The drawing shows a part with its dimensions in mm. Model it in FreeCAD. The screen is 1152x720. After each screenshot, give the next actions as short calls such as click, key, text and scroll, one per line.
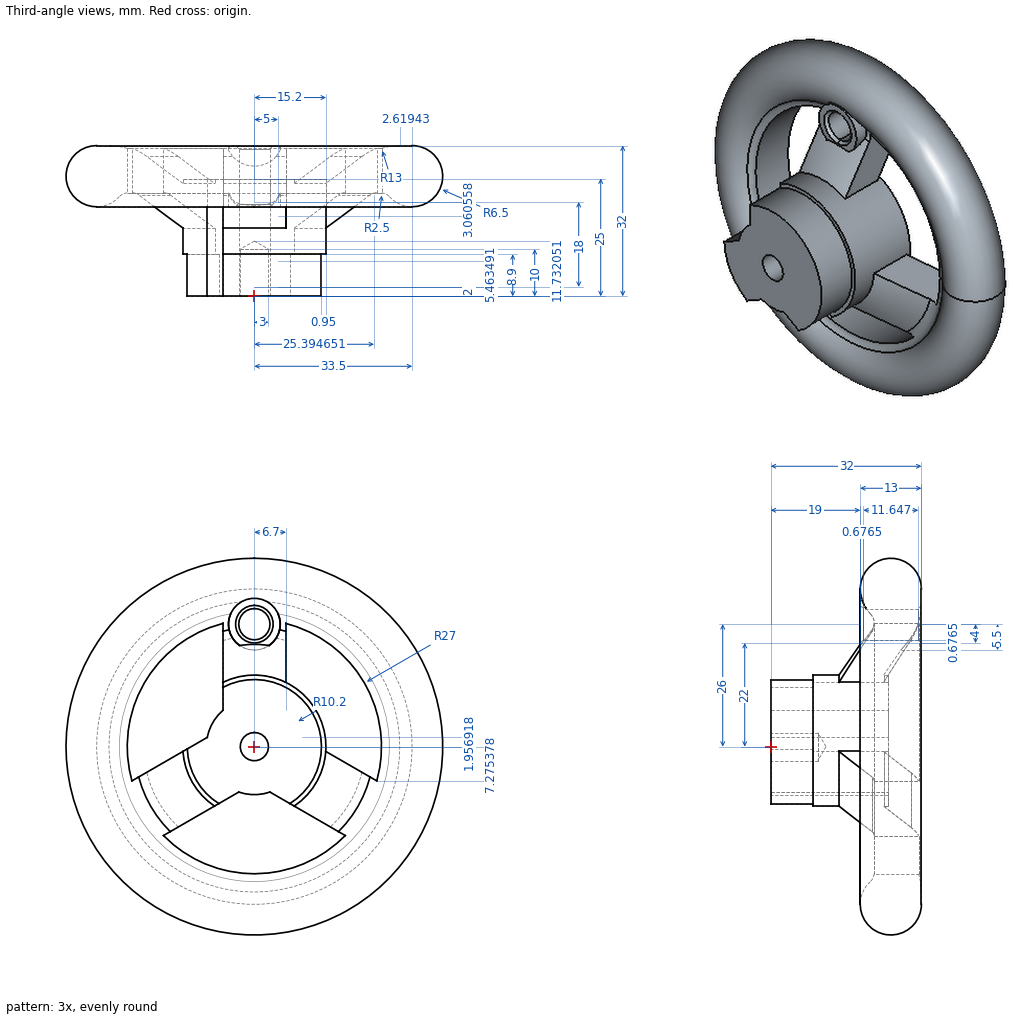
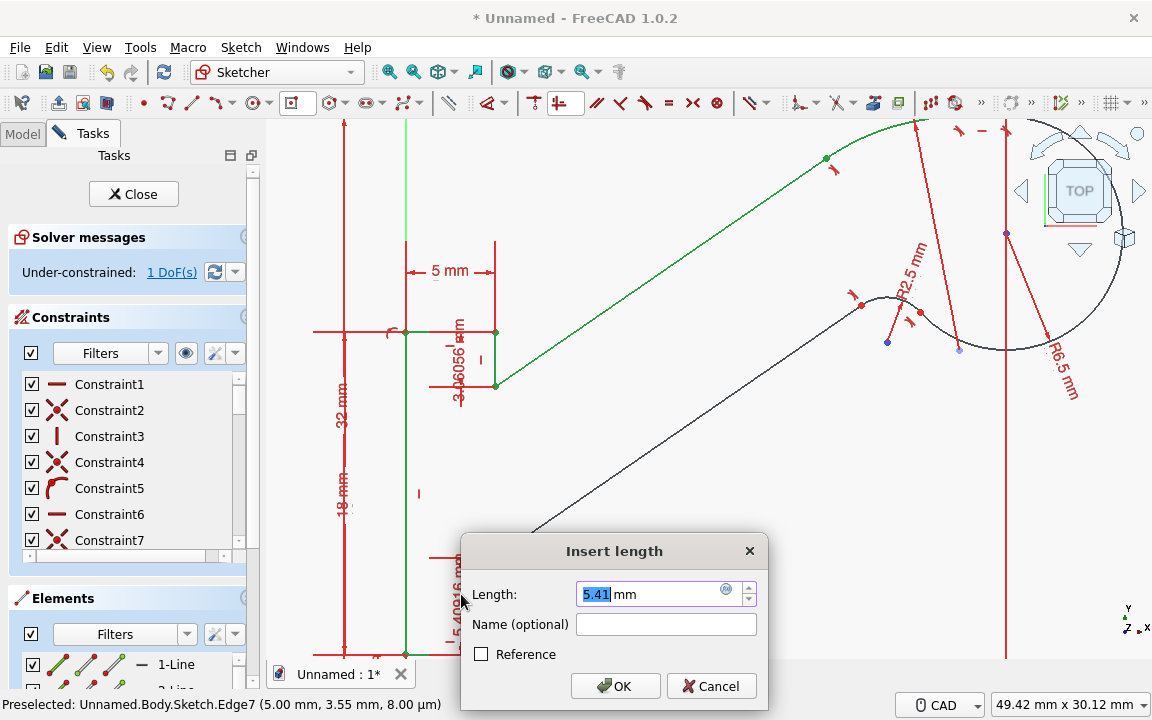
text(5.463491)
key(Return)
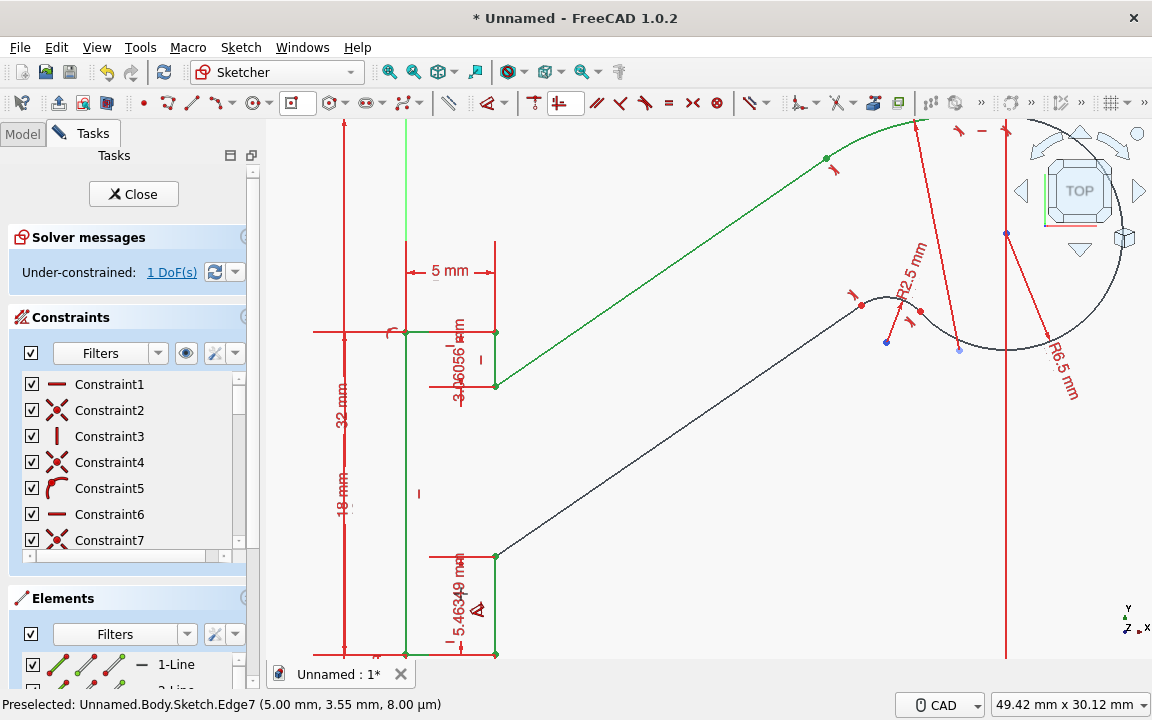
click(862, 305)
click(634, 271)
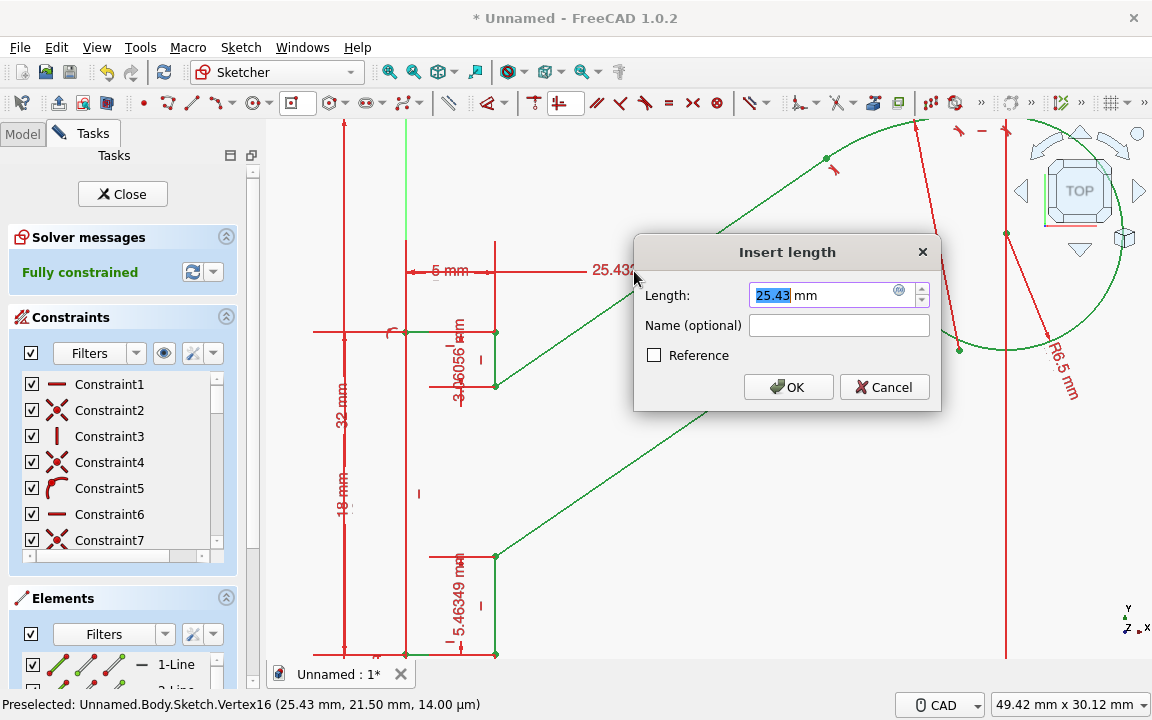
text(25.394651)
key(Return)
key(Escape)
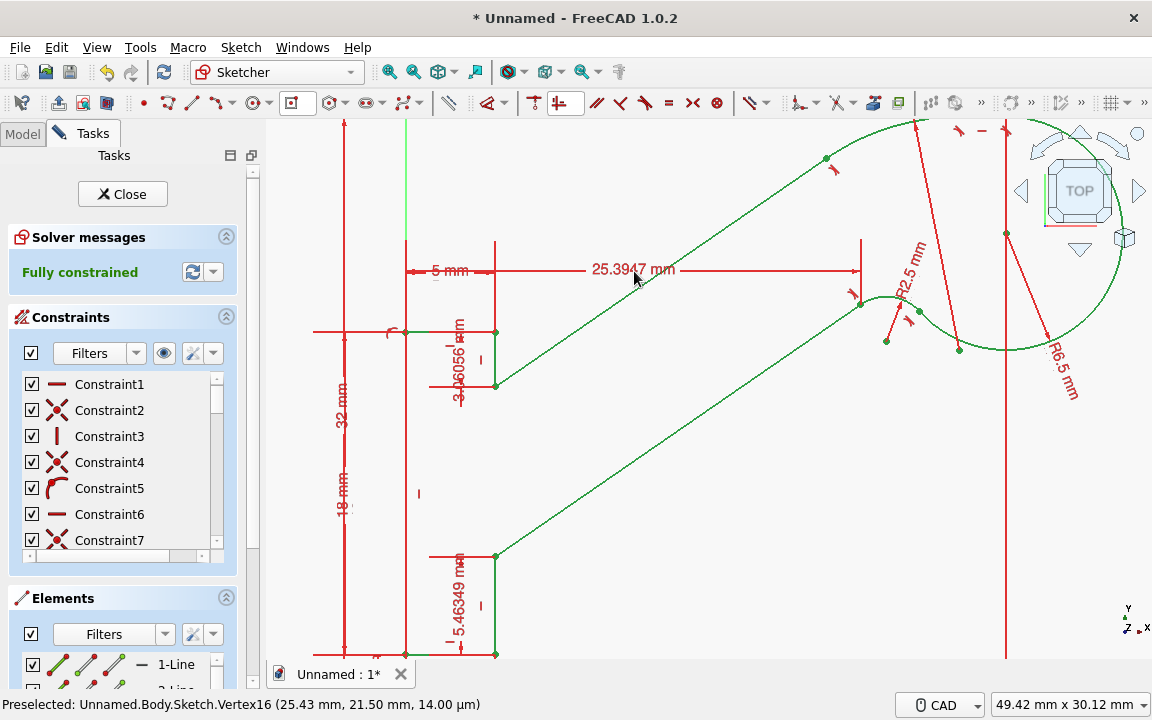
click(123, 194)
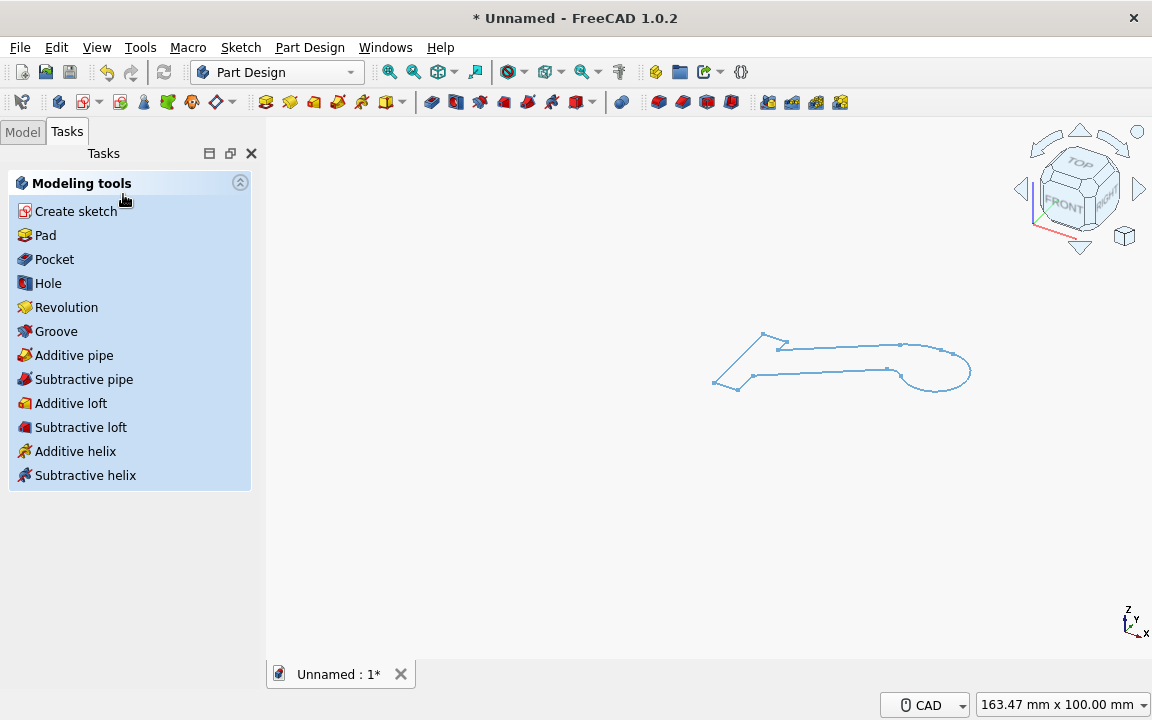
click(290, 102)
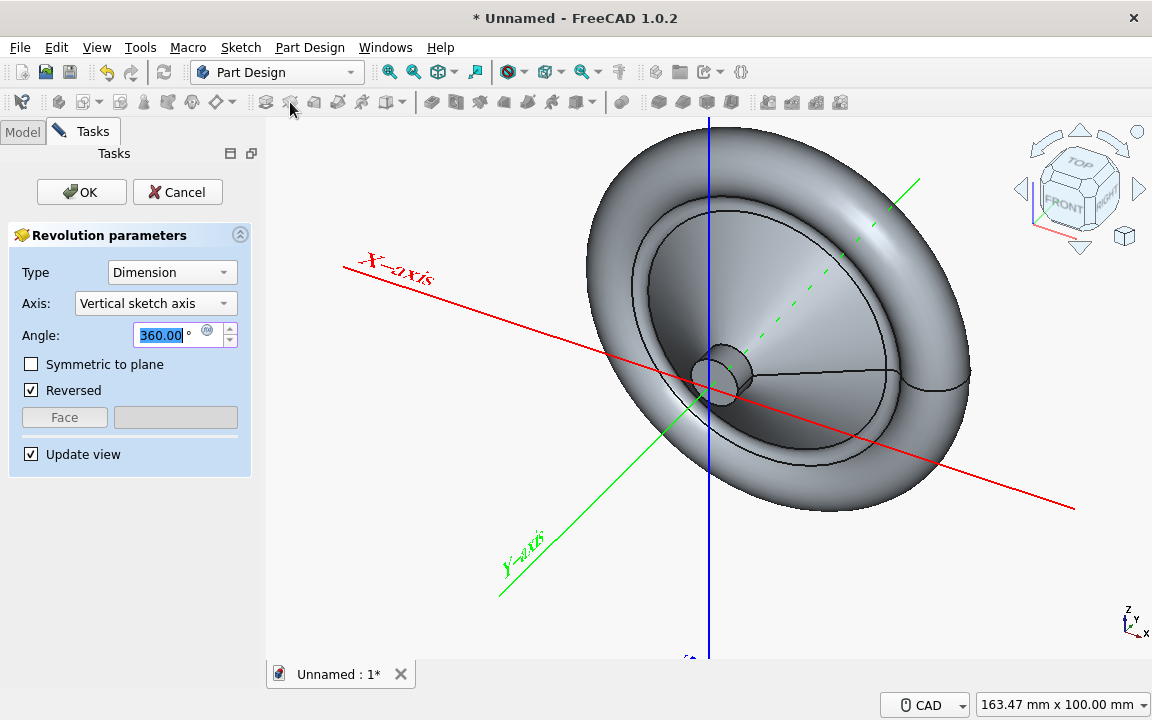
click(82, 192)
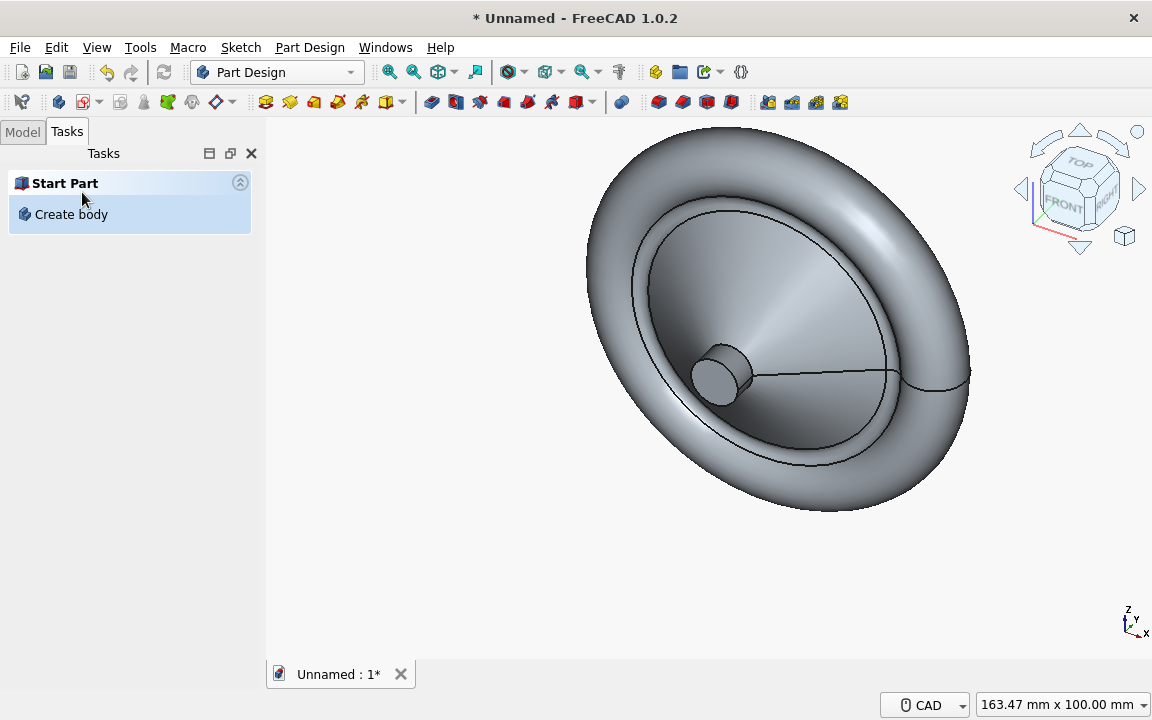
click(390, 72)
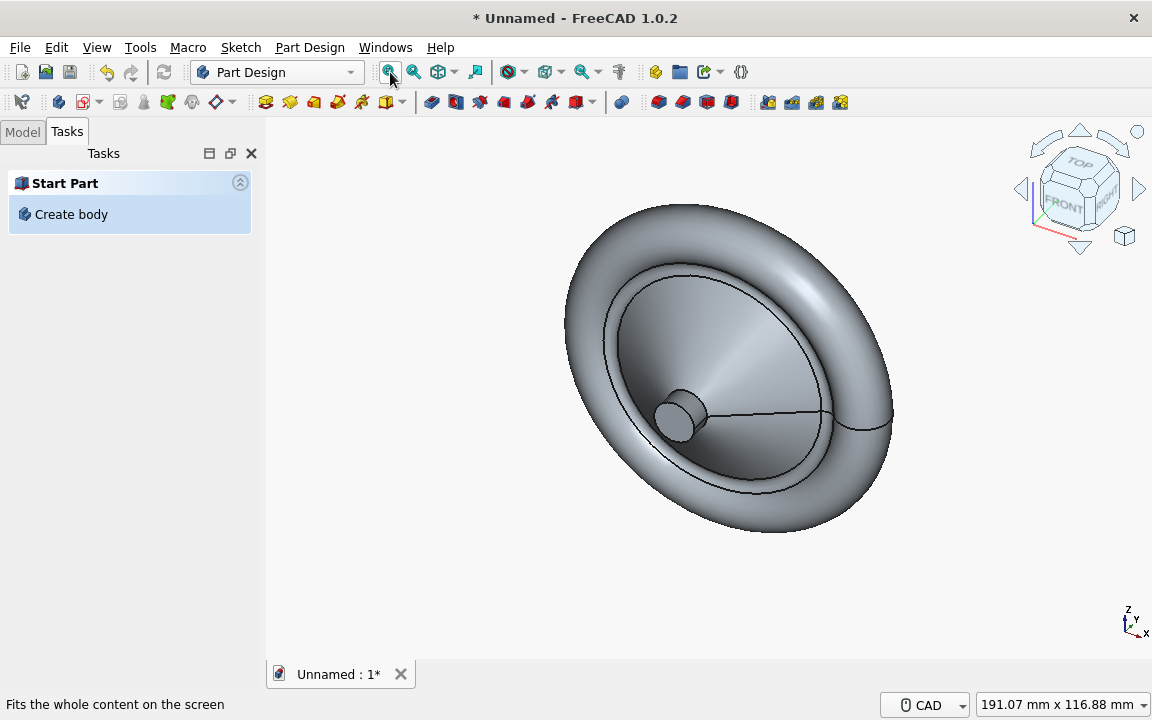
click(84, 102)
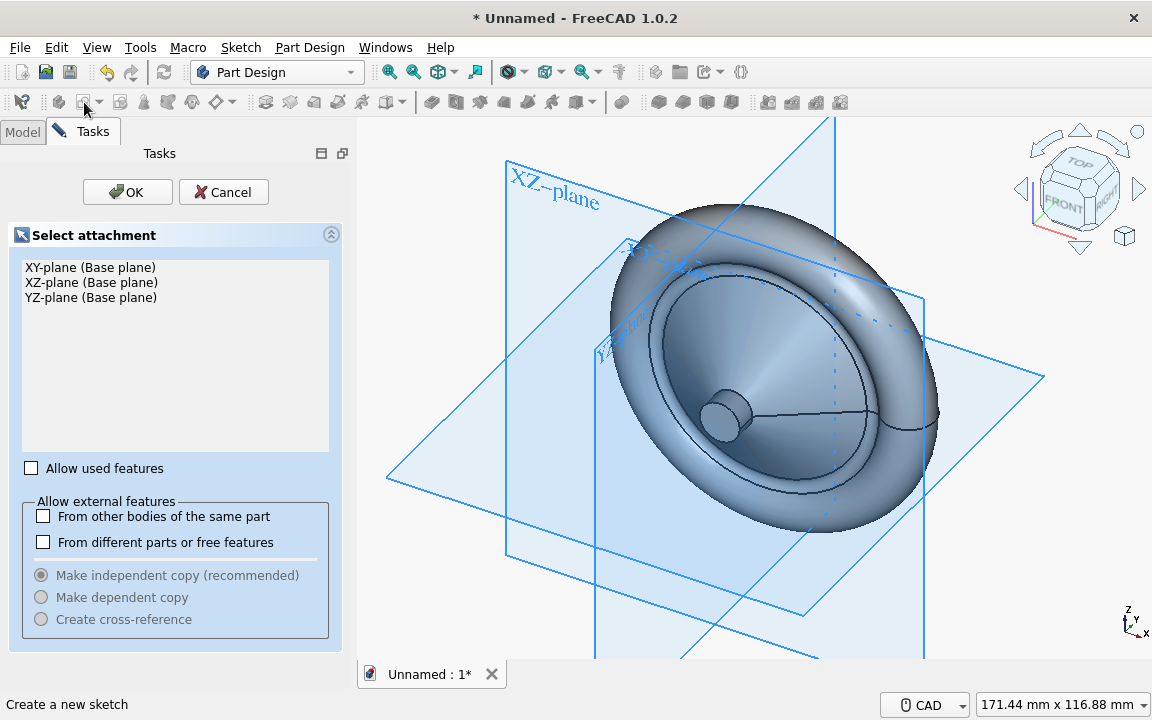
click(82, 282)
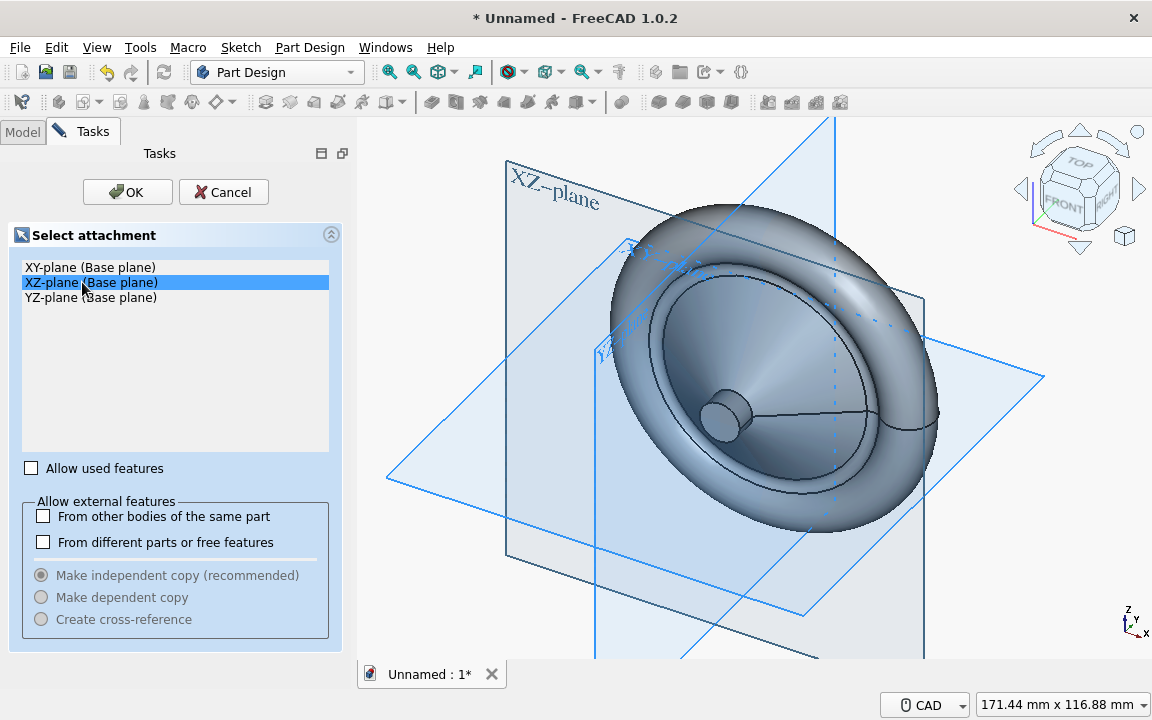
click(128, 192)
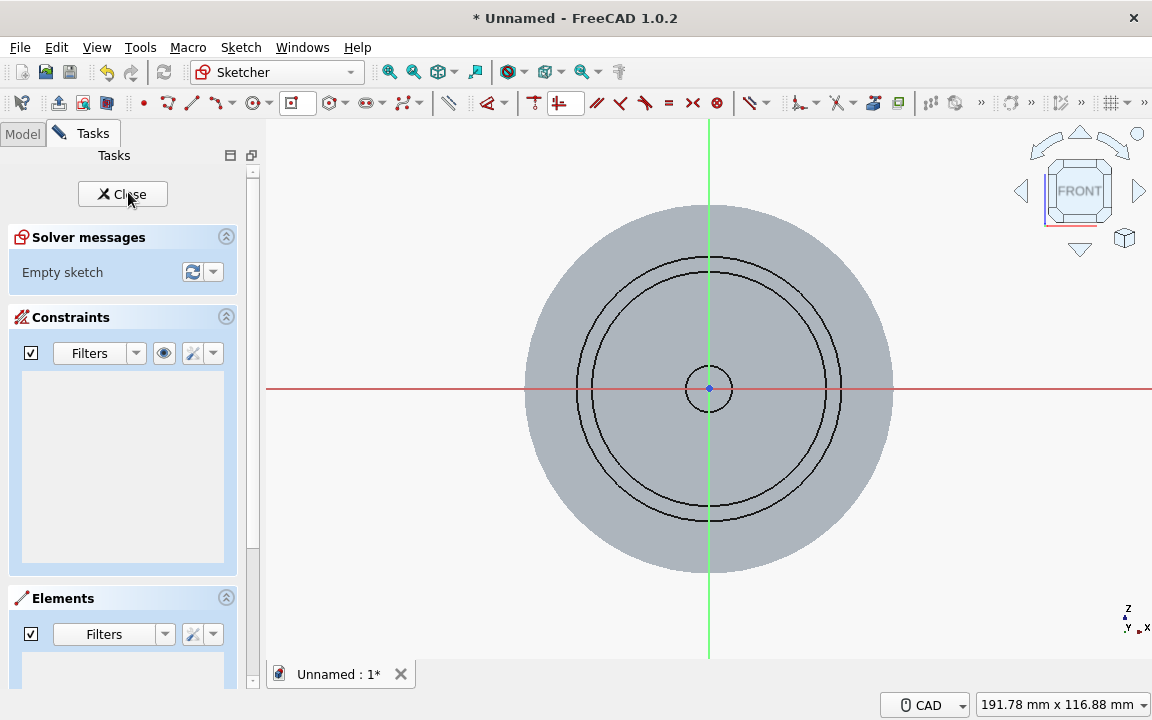
scroll(874, 310, up, 4)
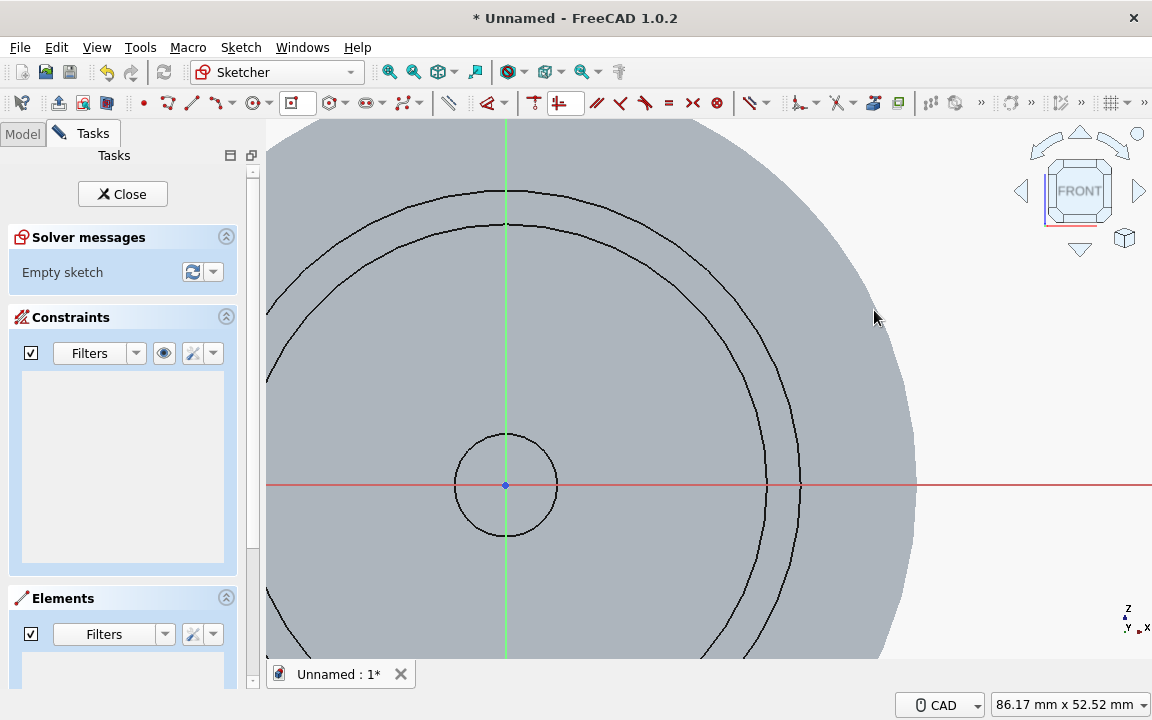
click(192, 104)